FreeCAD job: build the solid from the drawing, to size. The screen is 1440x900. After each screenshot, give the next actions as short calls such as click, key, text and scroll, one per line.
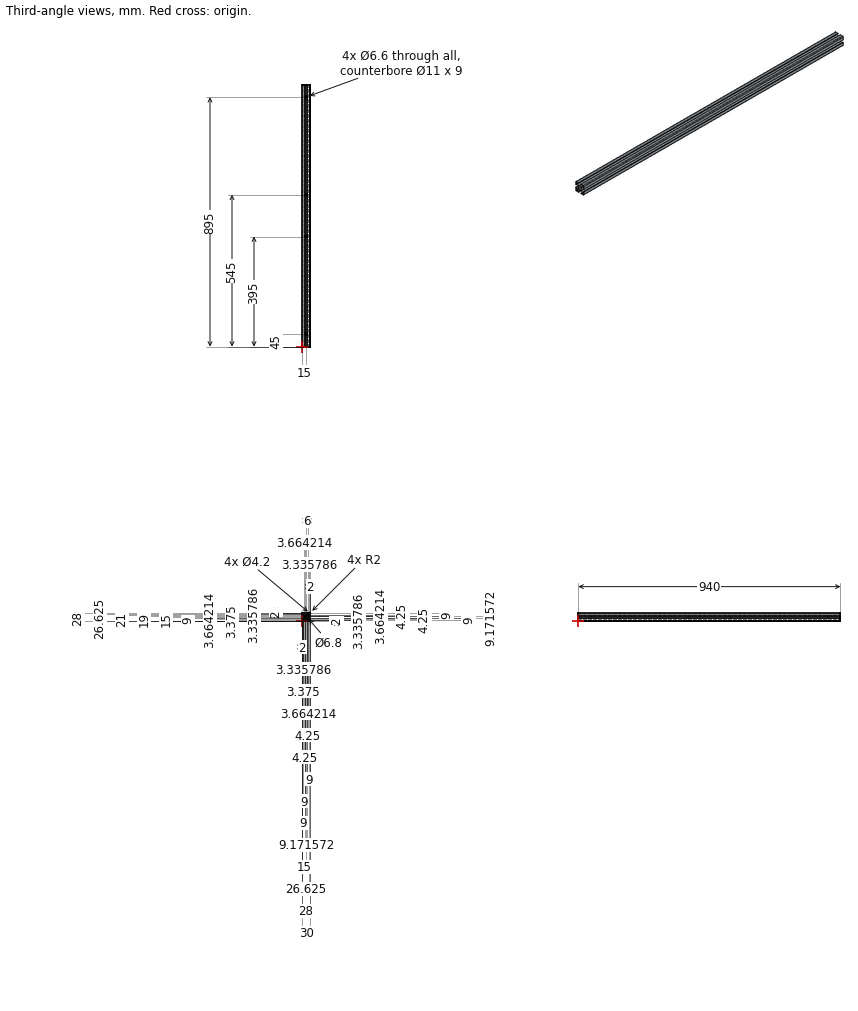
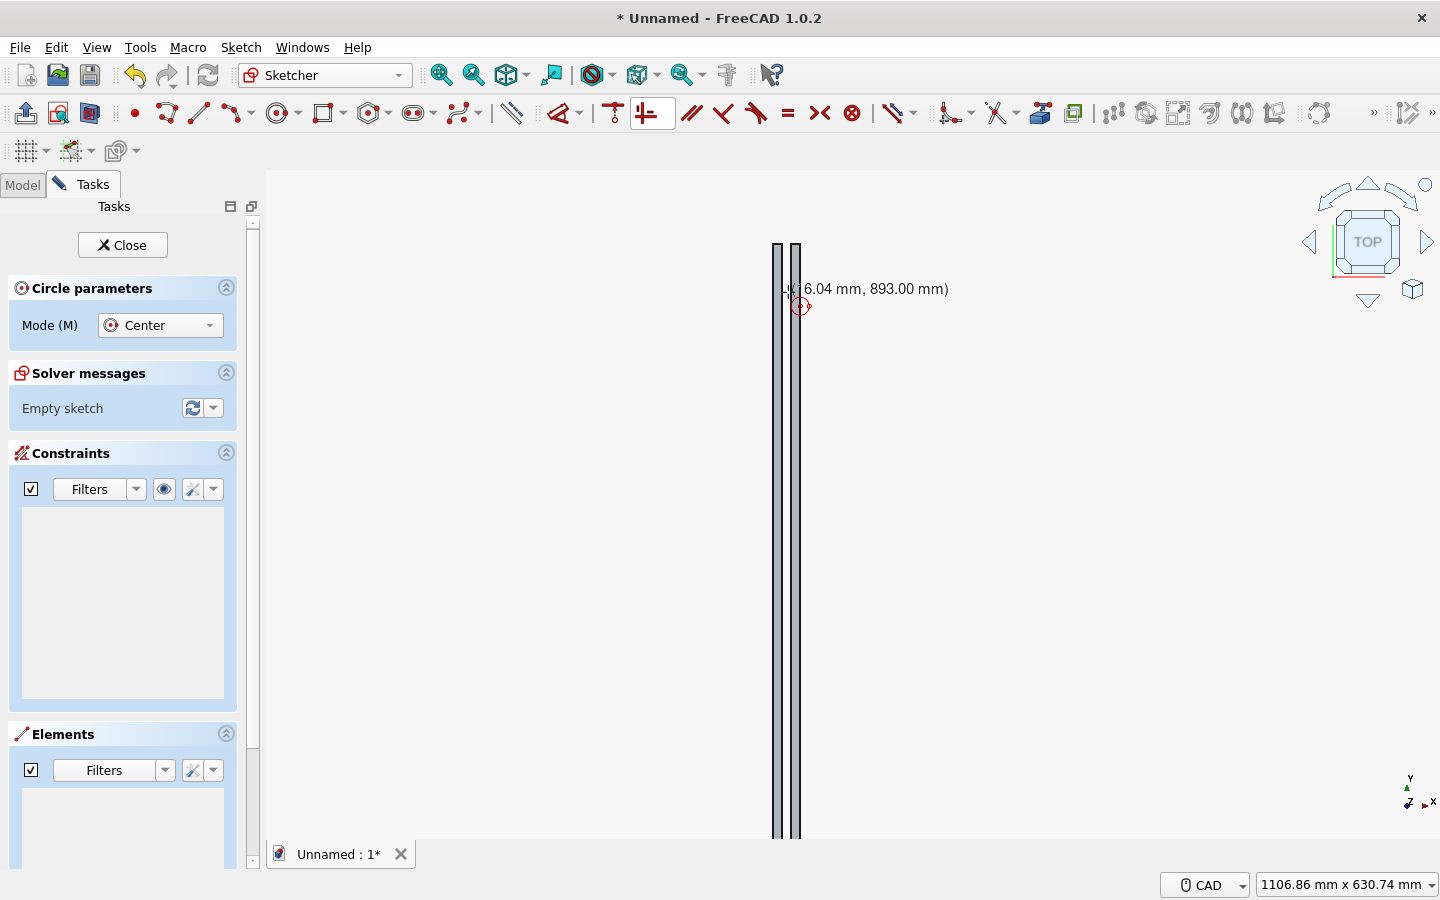
click(786, 292)
move(789, 289)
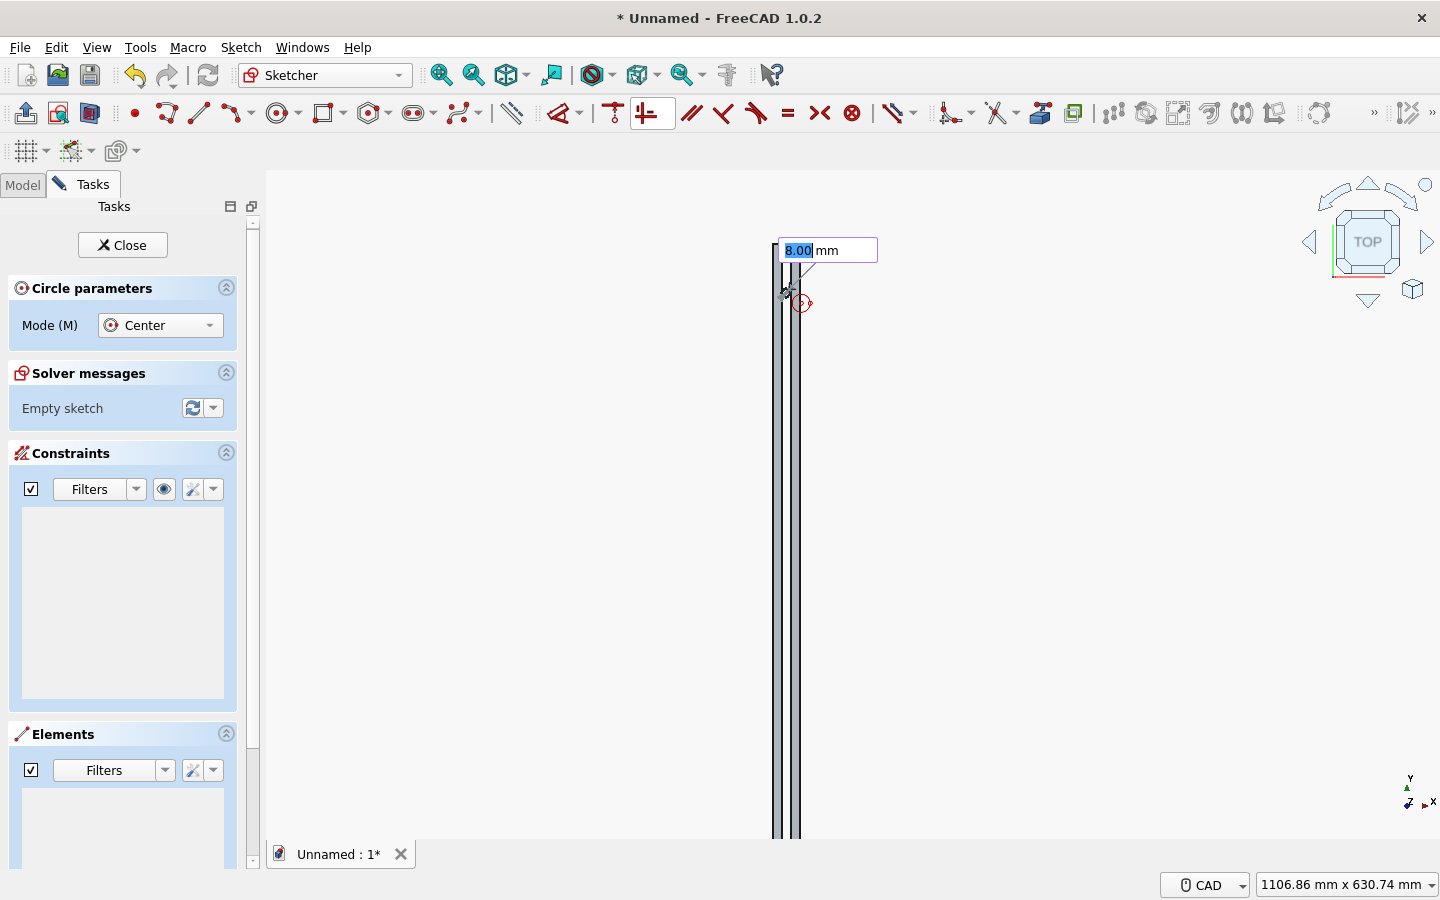
text(6.6)
key(Return)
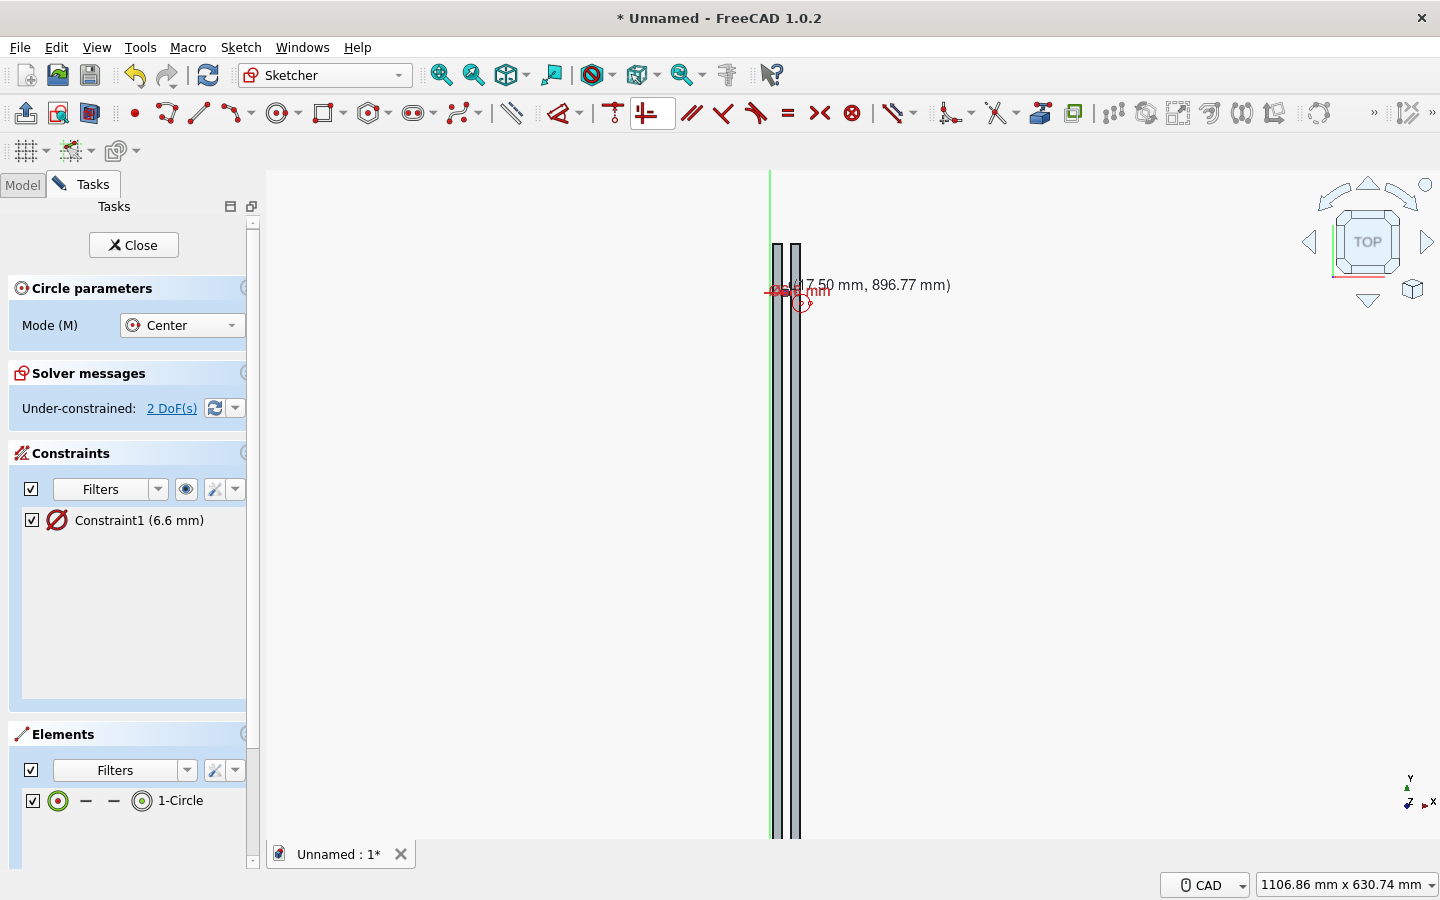
scroll(786, 663, up, 10)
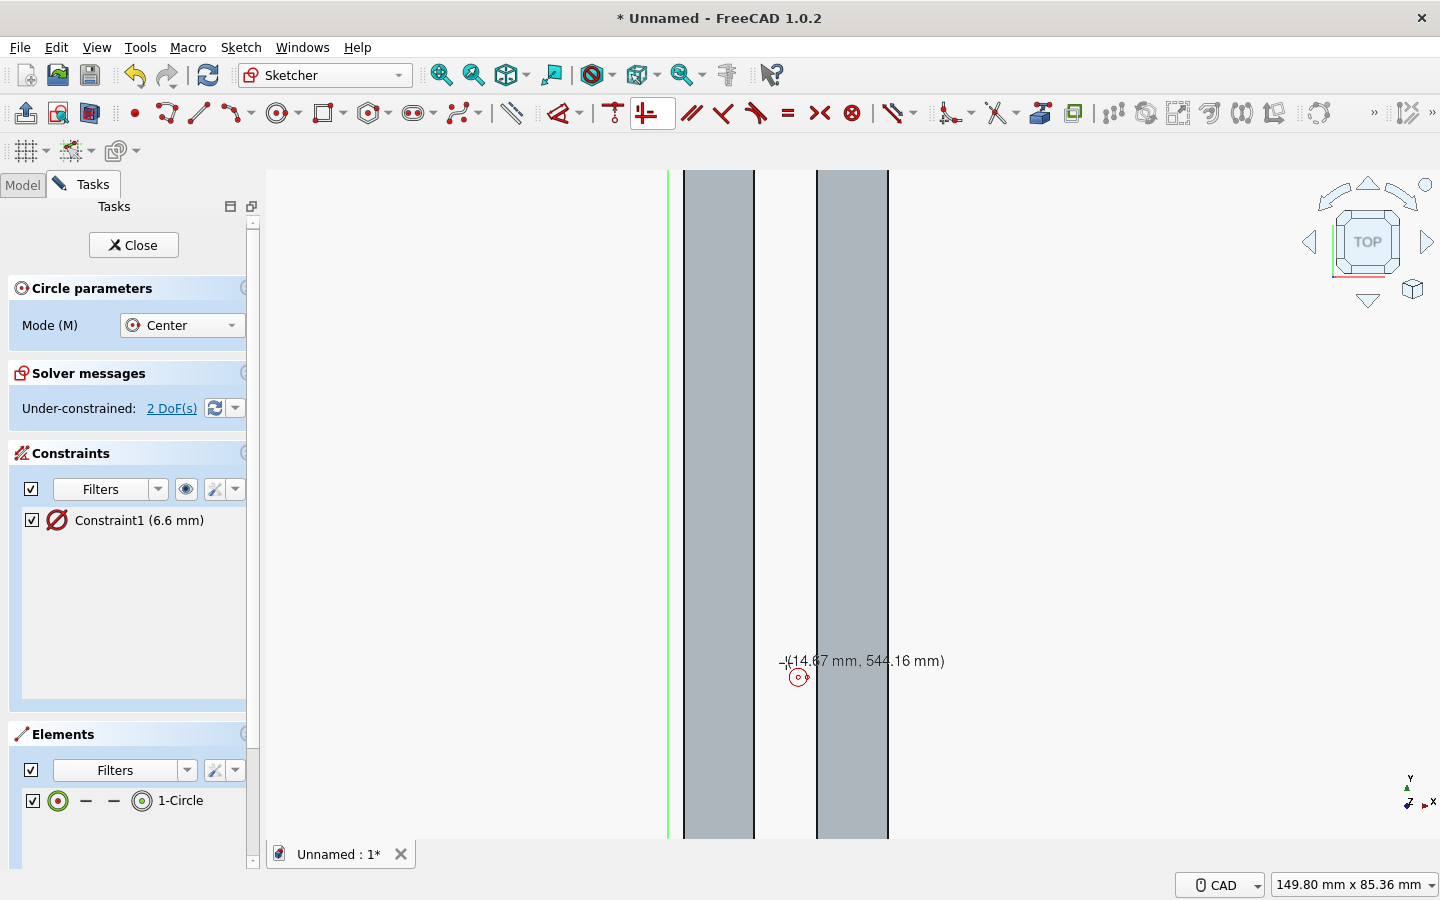
scroll(787, 446, down, 14)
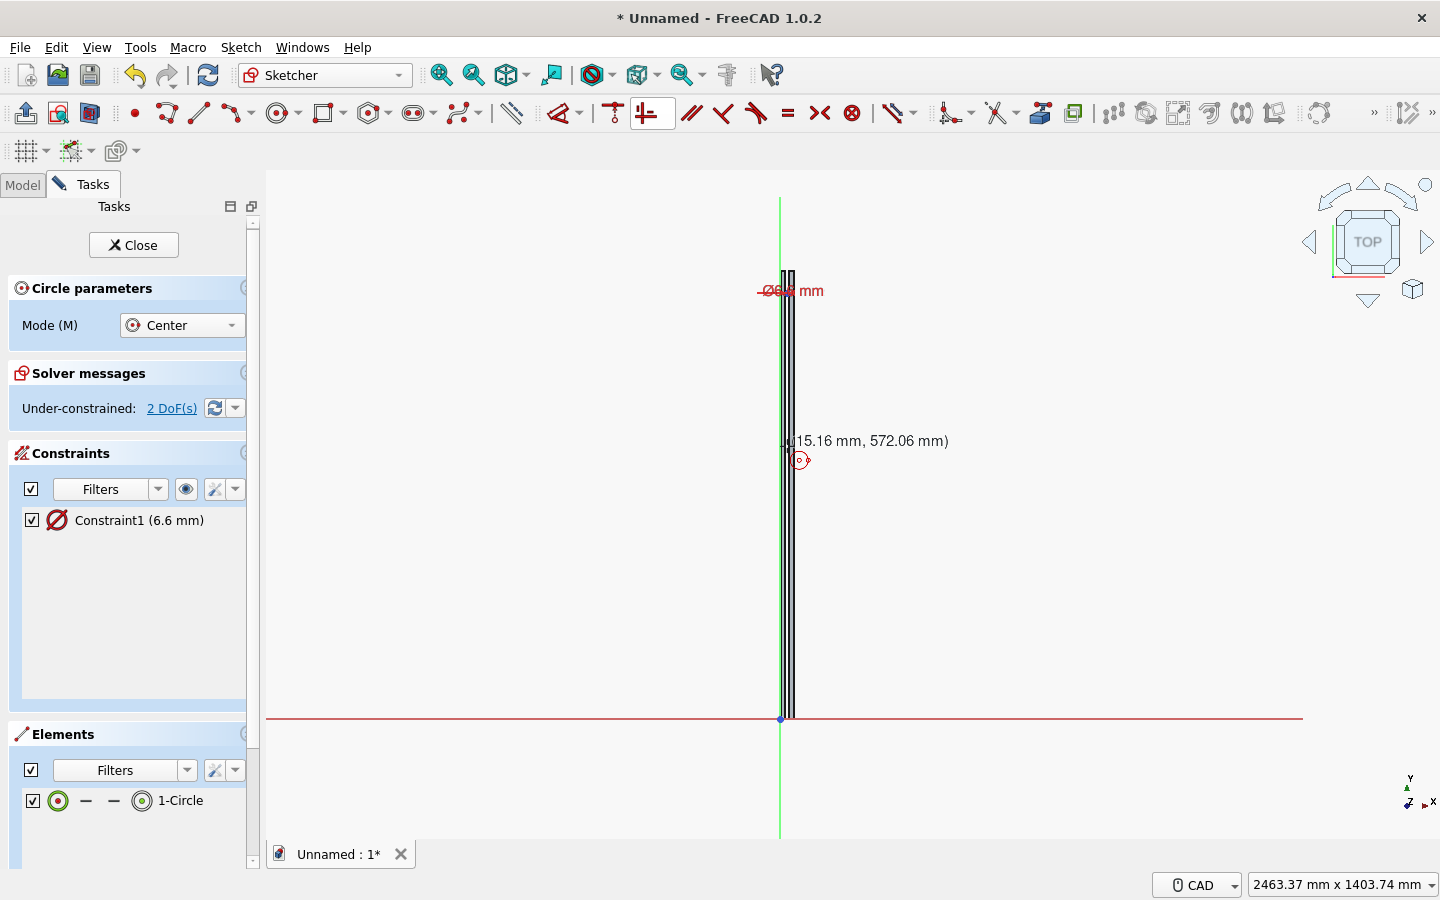
scroll(787, 459, up, 4)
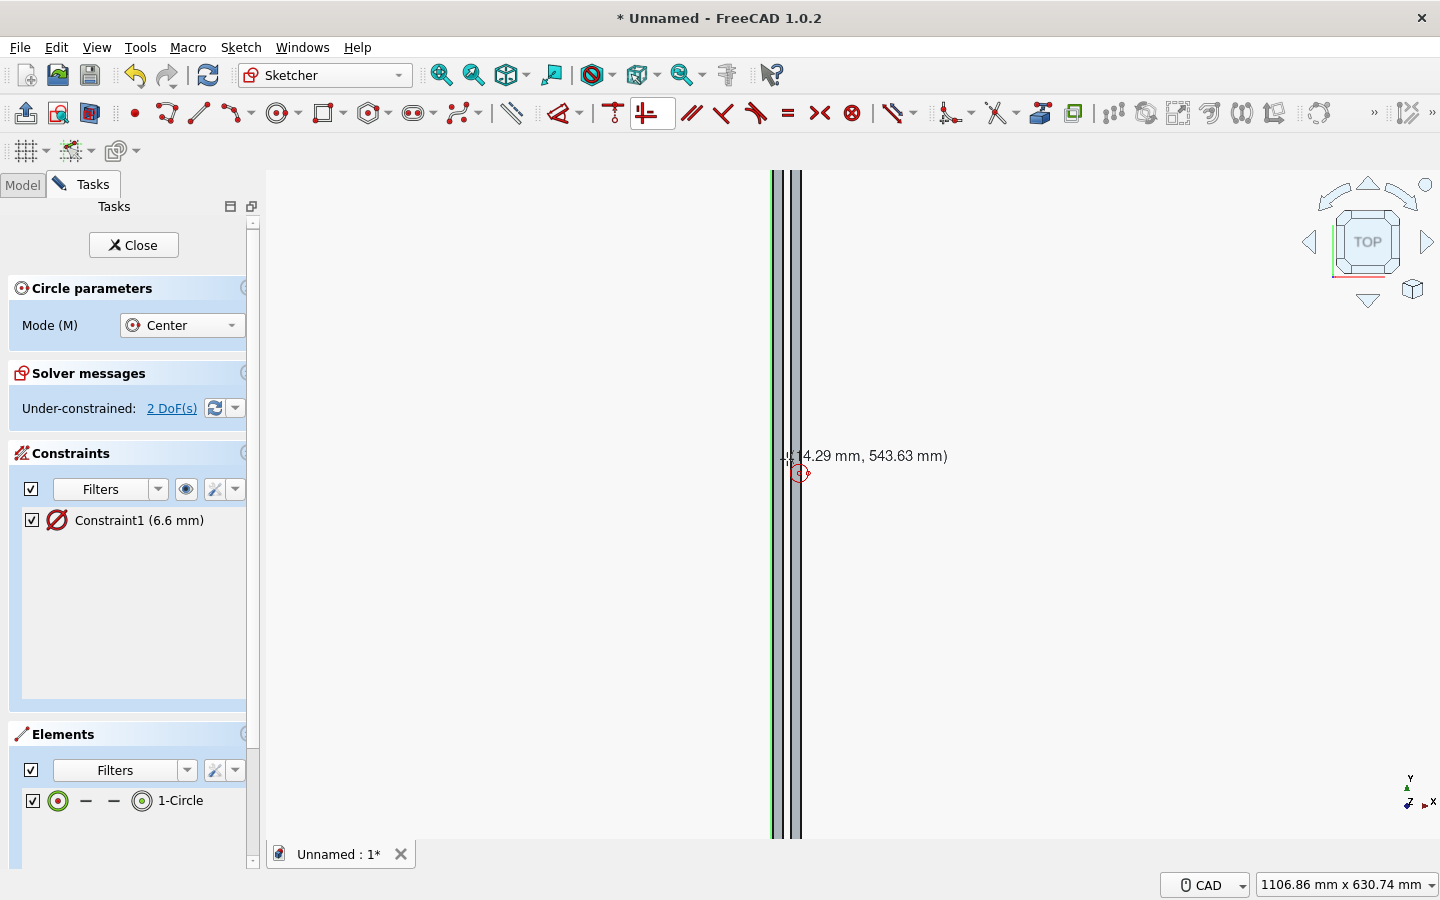
click(787, 459)
move(790, 457)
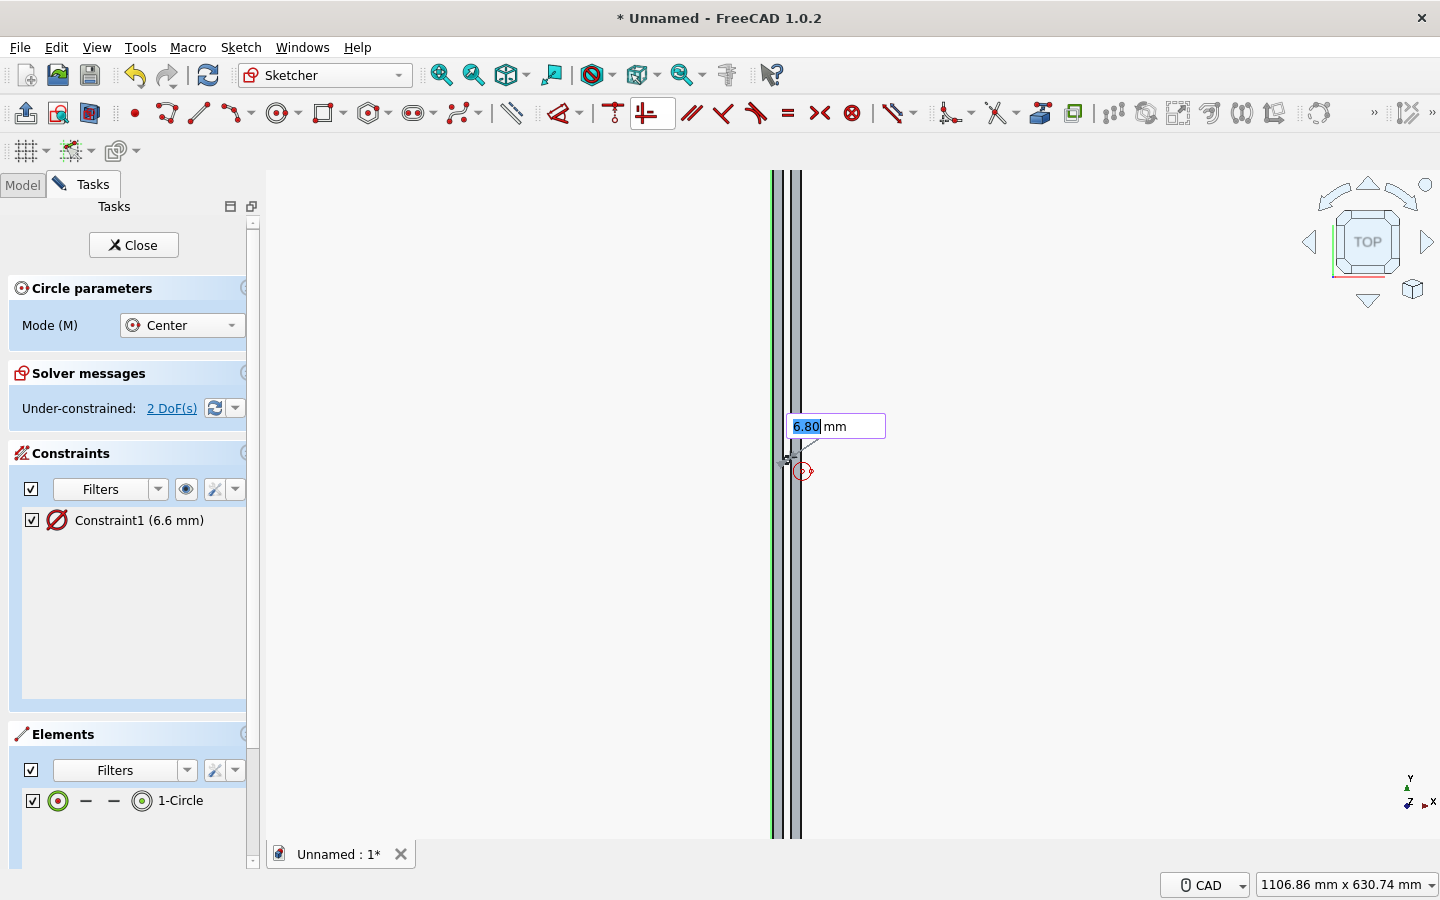
text(6.6)
key(Return)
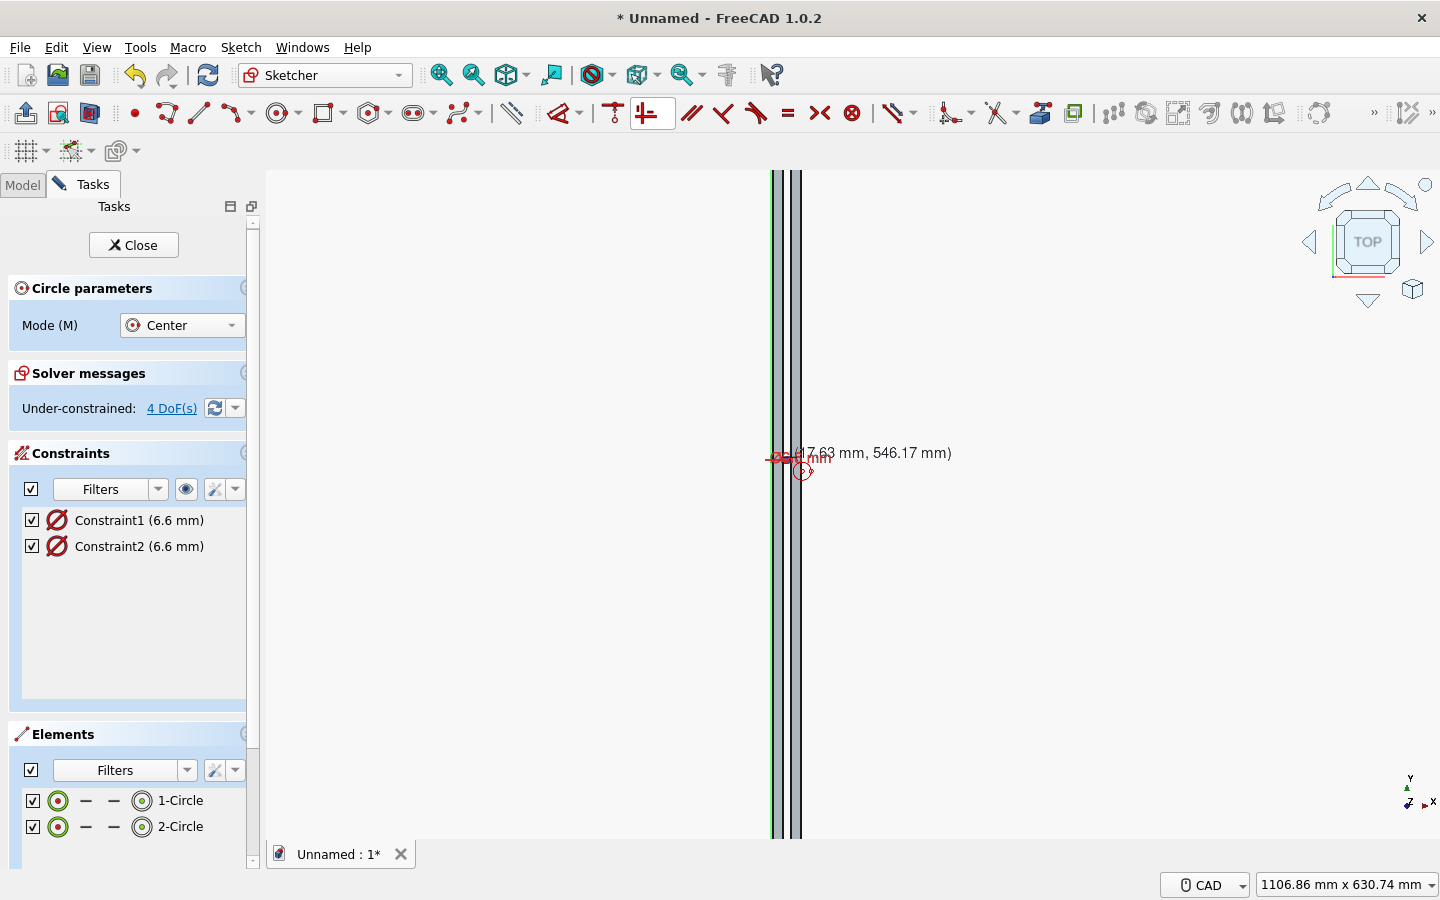
scroll(787, 458, down, 4)